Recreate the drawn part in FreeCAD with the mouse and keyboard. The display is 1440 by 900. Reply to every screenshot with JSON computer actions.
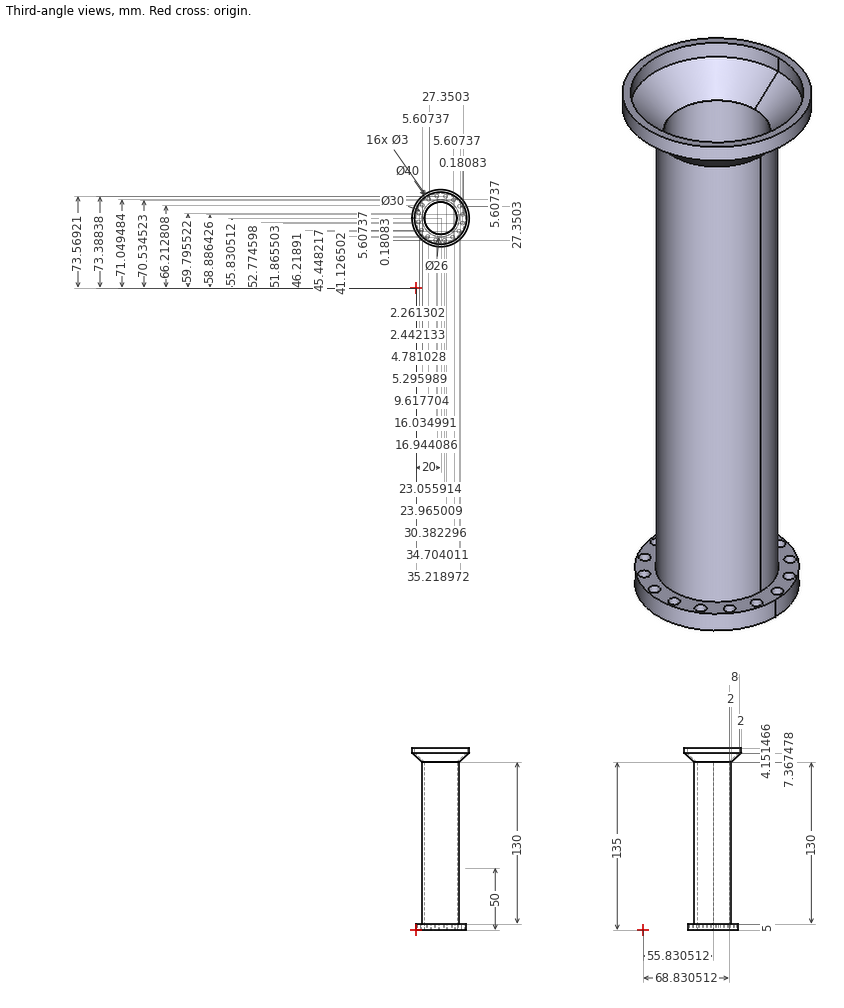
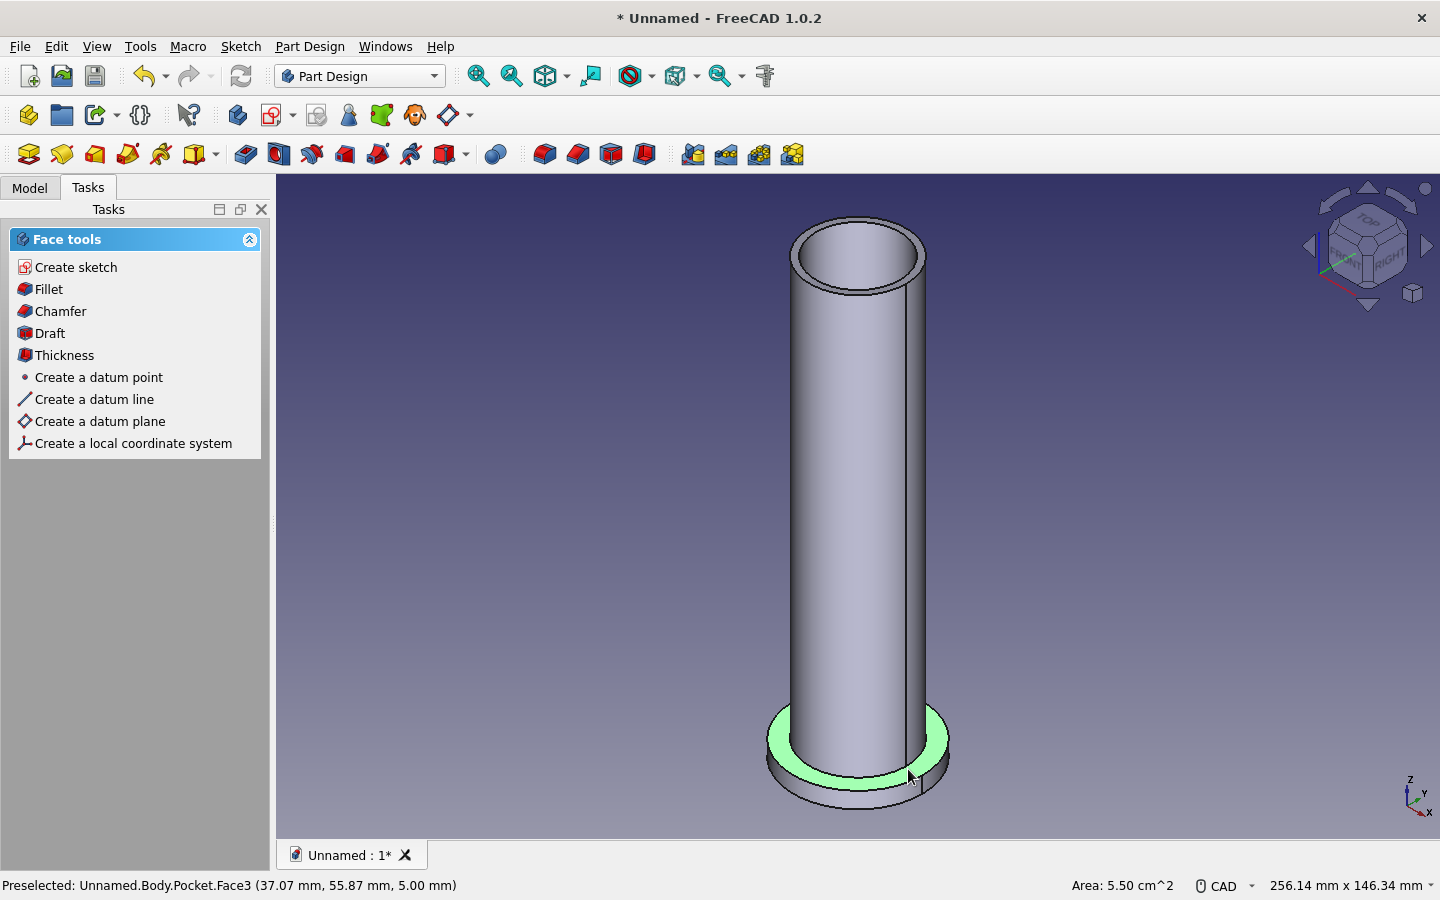
{"action": "left_click", "coordinate": [270, 116]}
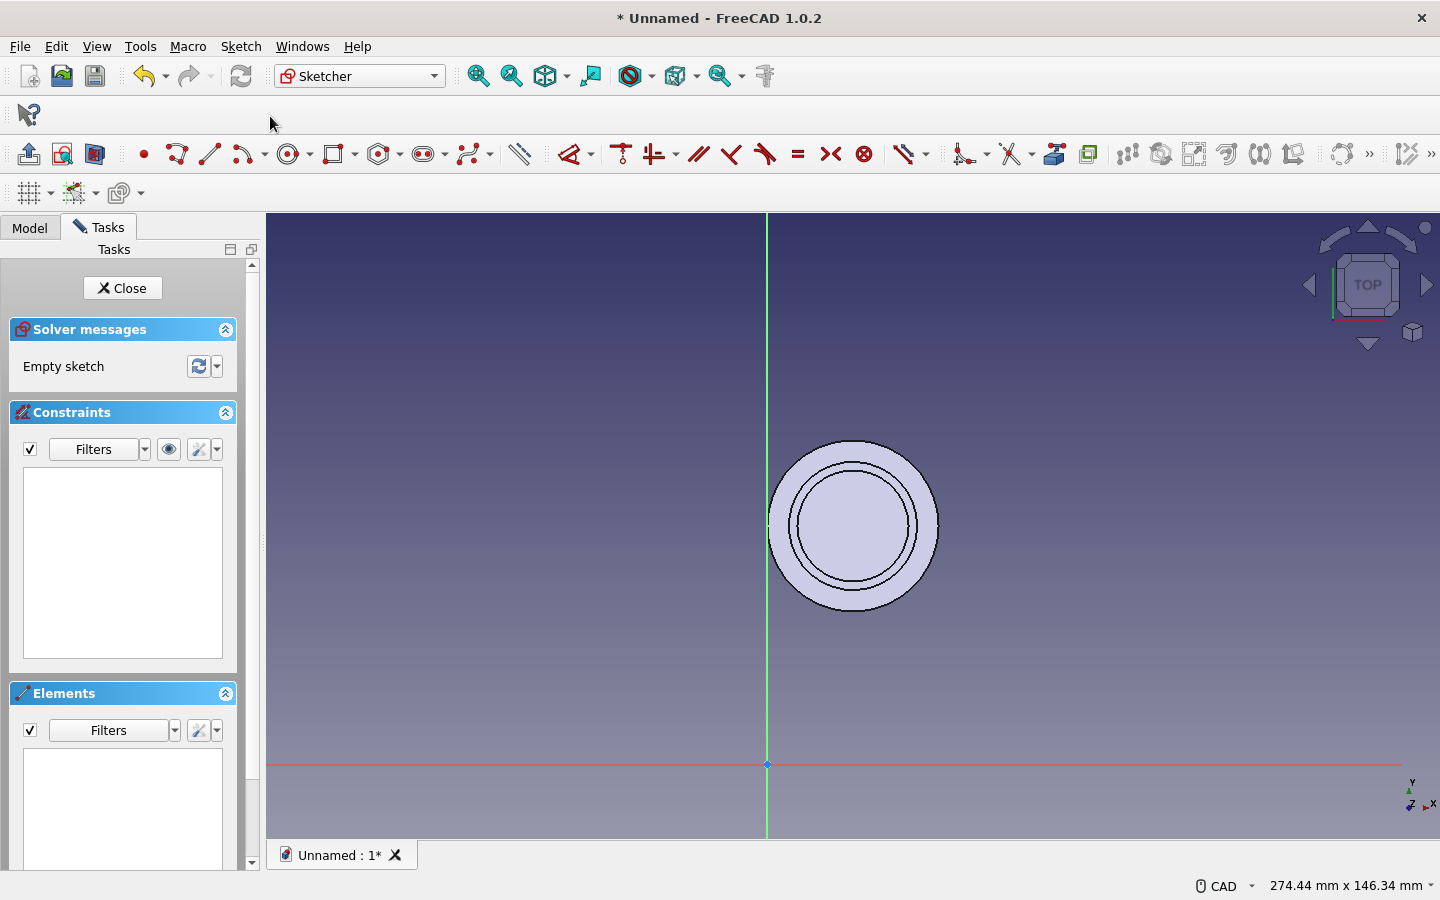
{"action": "left_click", "coordinate": [95, 154]}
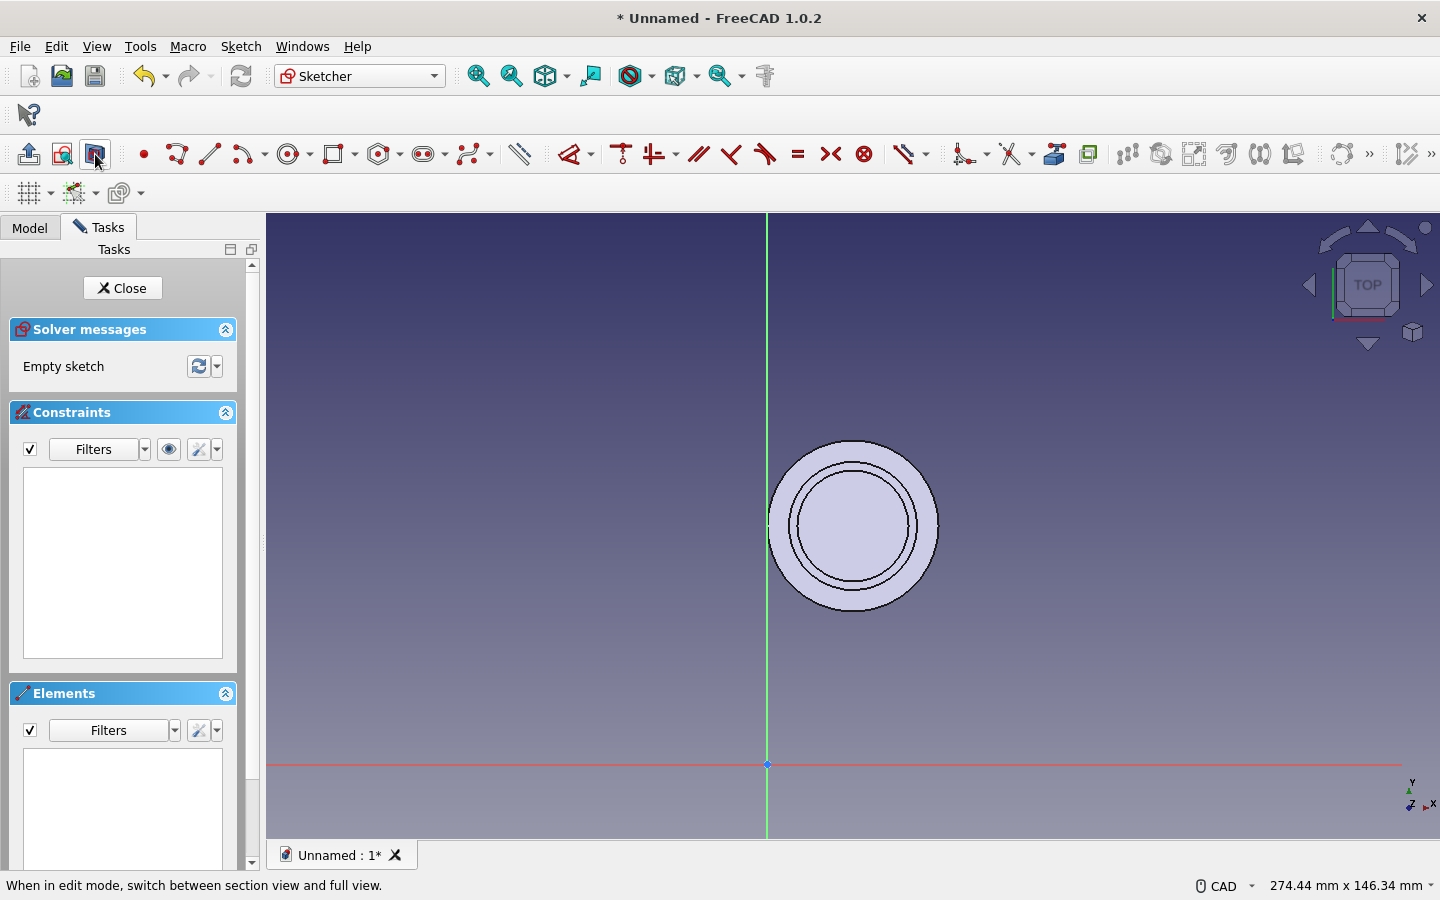
{"action": "scroll", "coordinate": [883, 526], "scroll_direction": "up", "scroll_amount": 6}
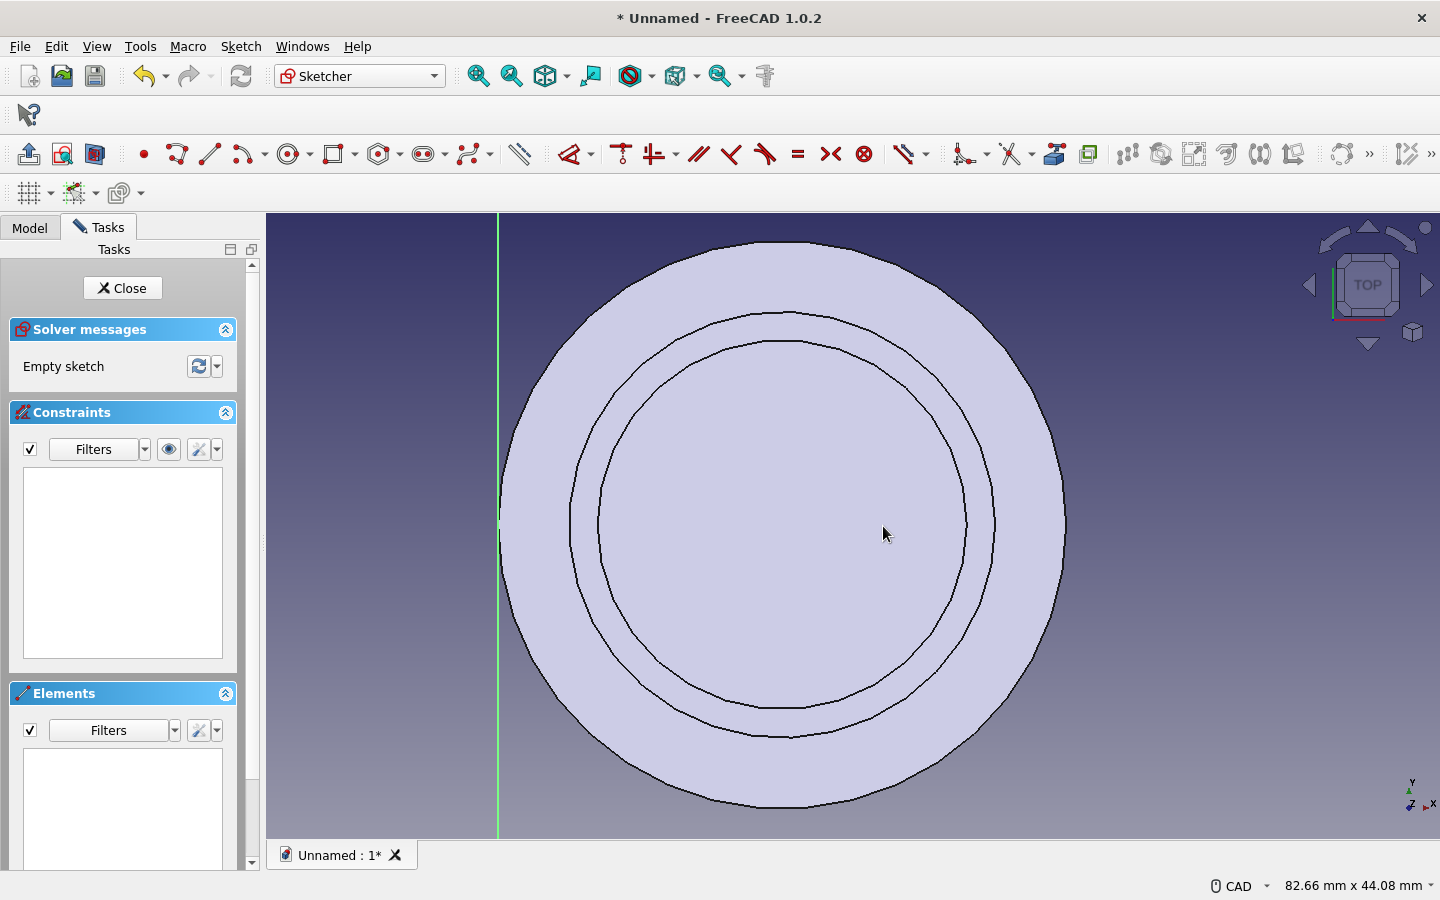
{"action": "key", "text": "g c"}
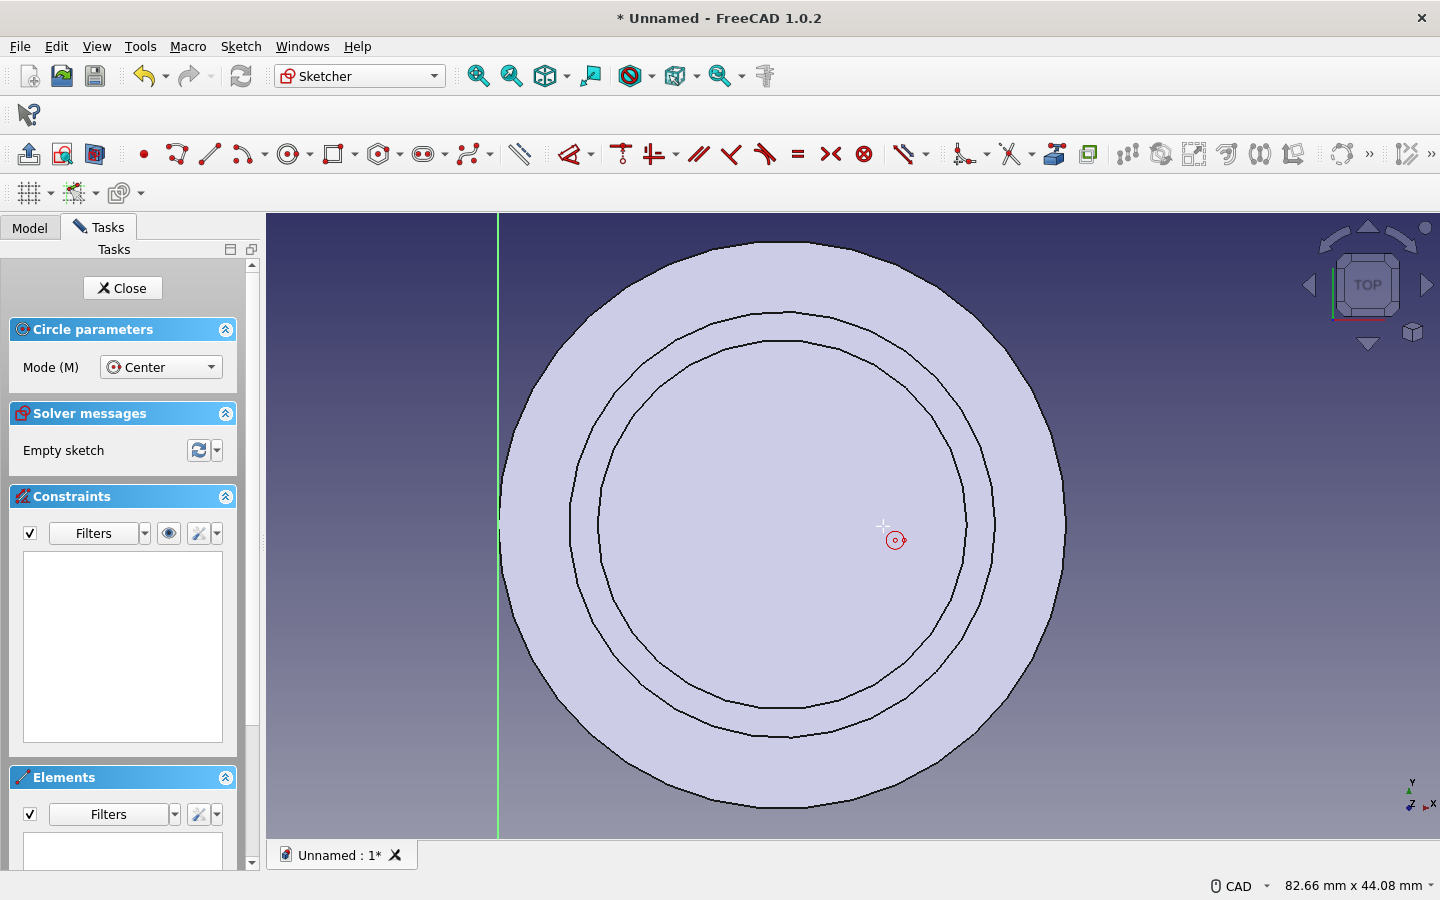
{"action": "left_click", "coordinate": [782, 525]}
{"action": "mouse_move", "coordinate": [913, 394]}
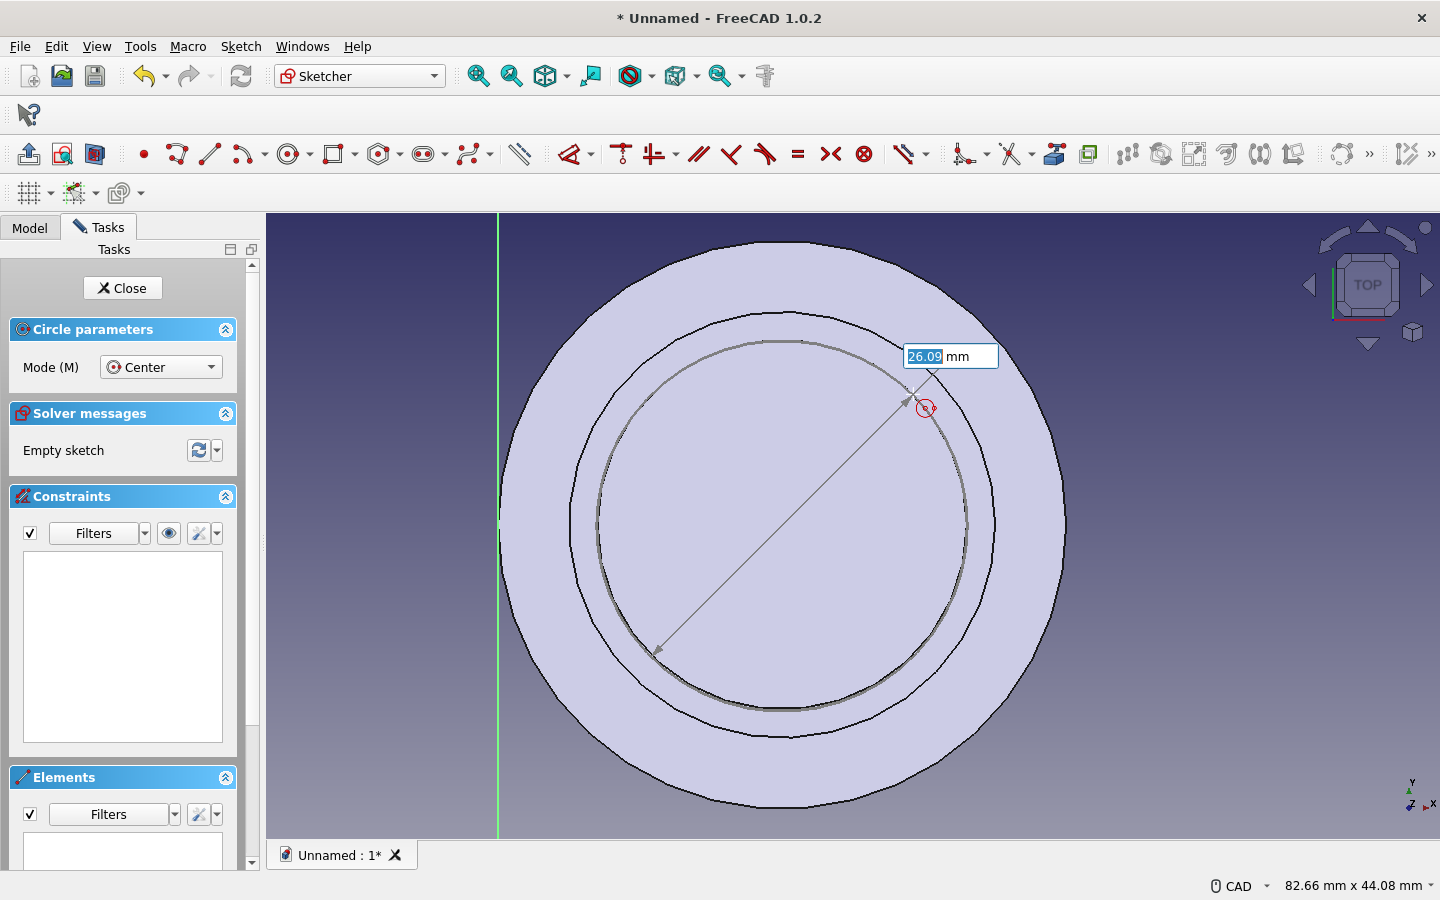
{"action": "type", "text": "26"}
{"action": "key", "text": "Return"}
{"action": "key", "text": "Escape"}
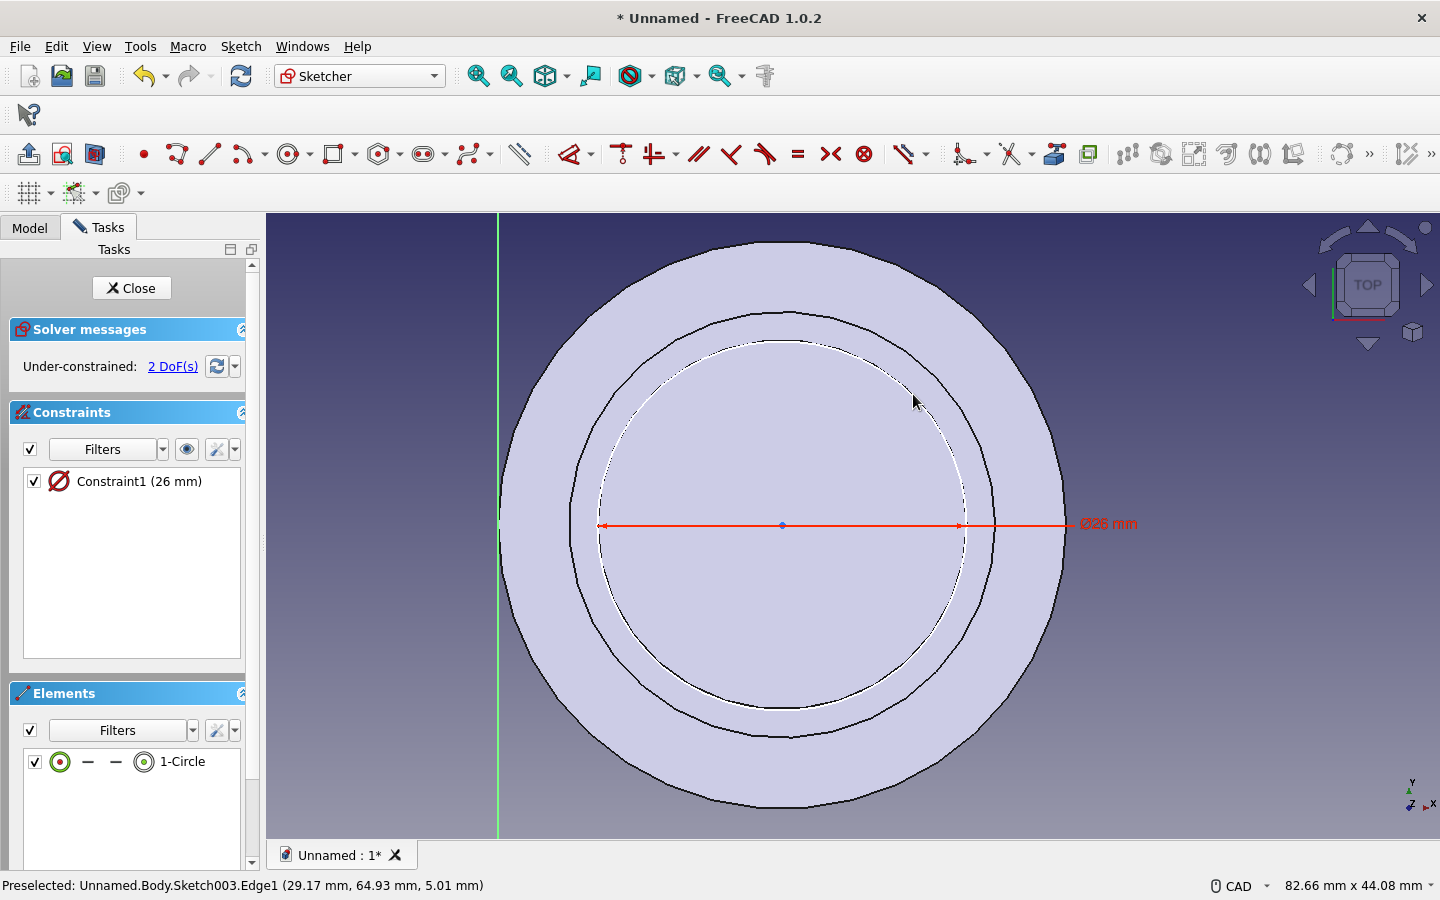
{"action": "left_click", "coordinate": [568, 154]}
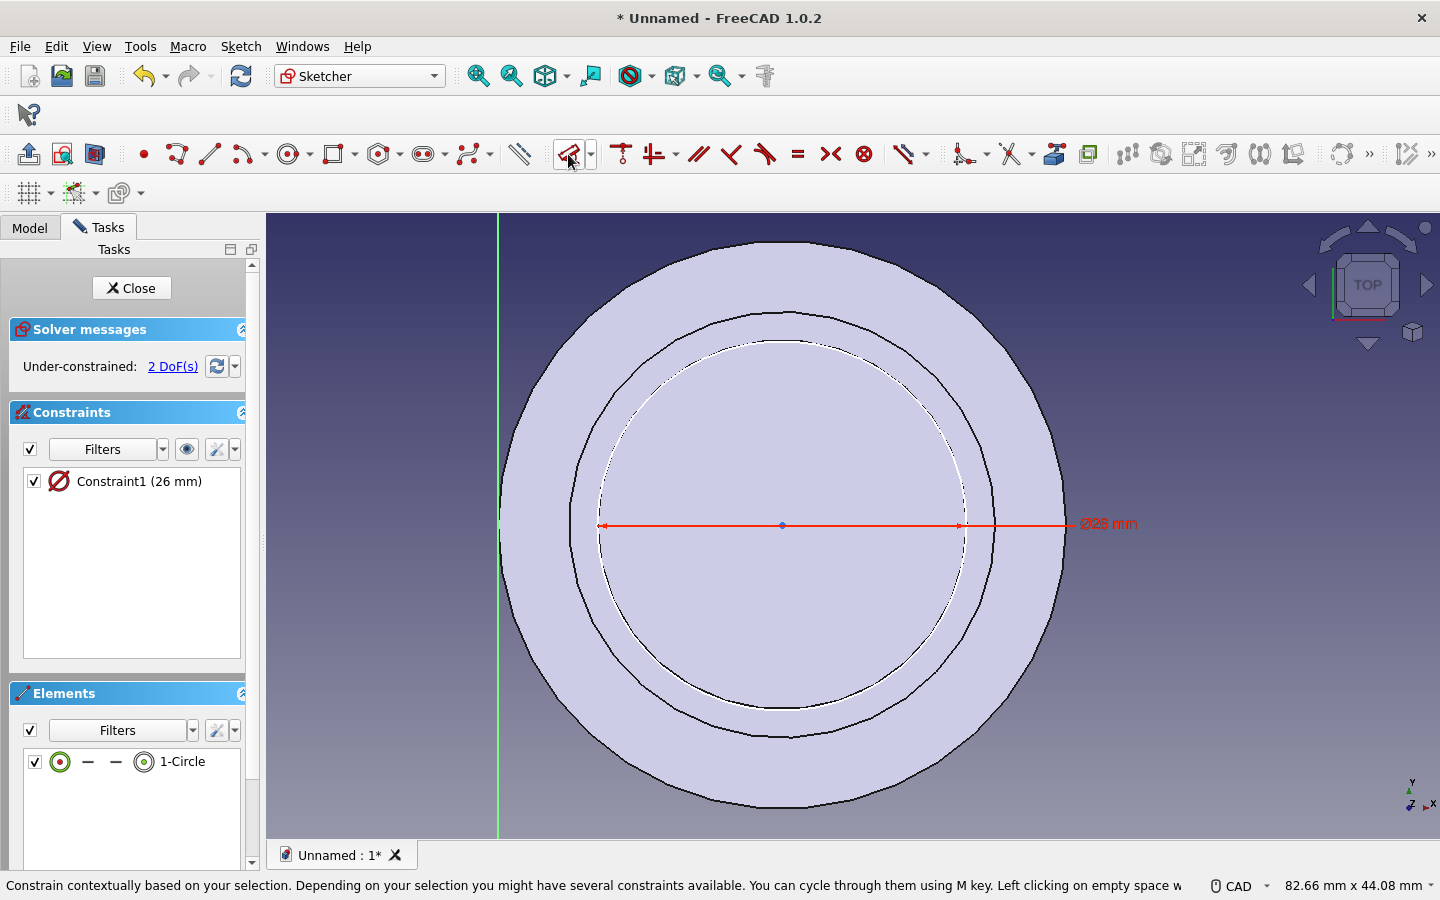
{"action": "left_click", "coordinate": [782, 526]}
{"action": "left_click", "coordinate": [640, 492]}